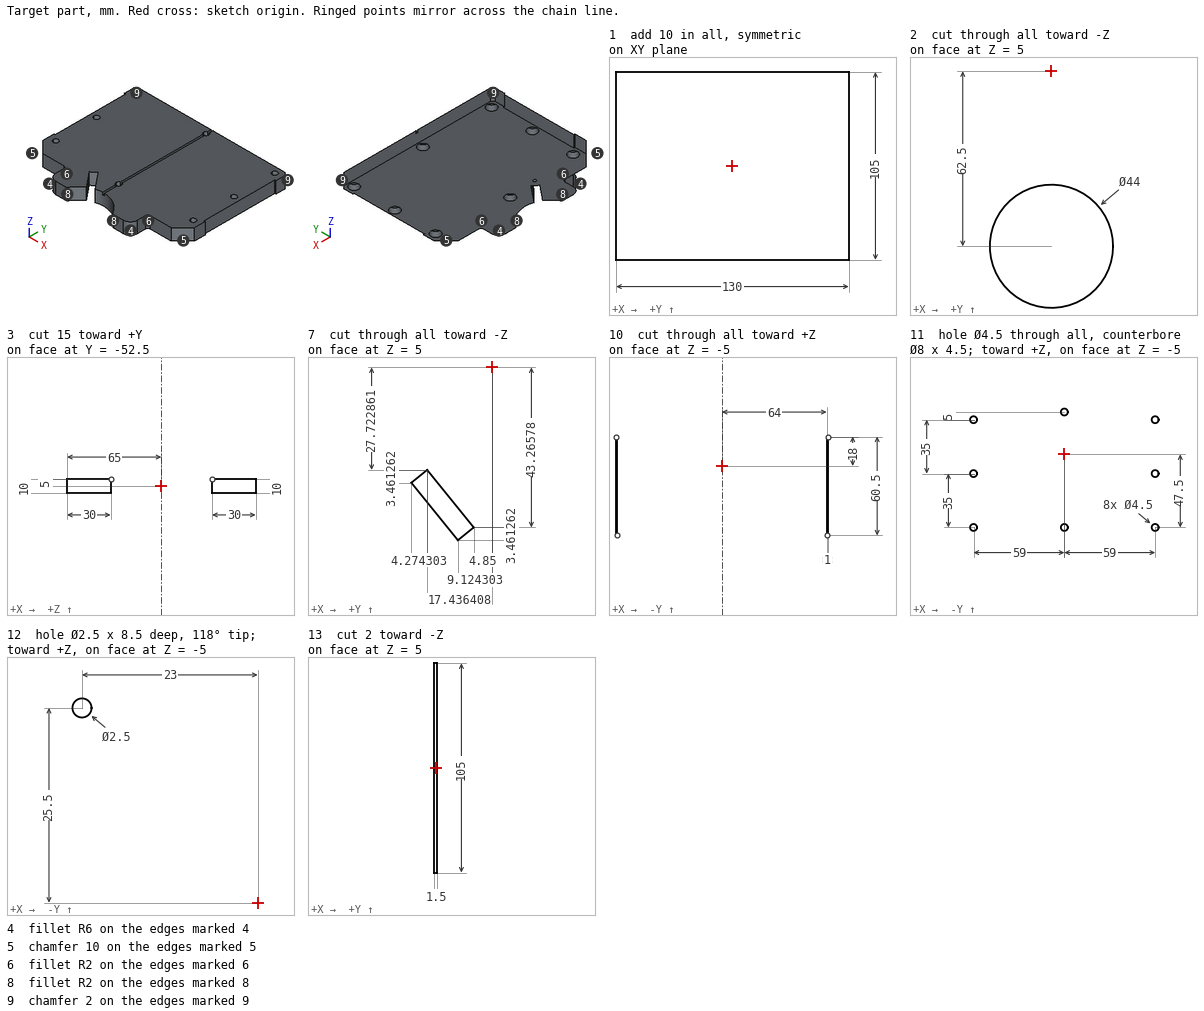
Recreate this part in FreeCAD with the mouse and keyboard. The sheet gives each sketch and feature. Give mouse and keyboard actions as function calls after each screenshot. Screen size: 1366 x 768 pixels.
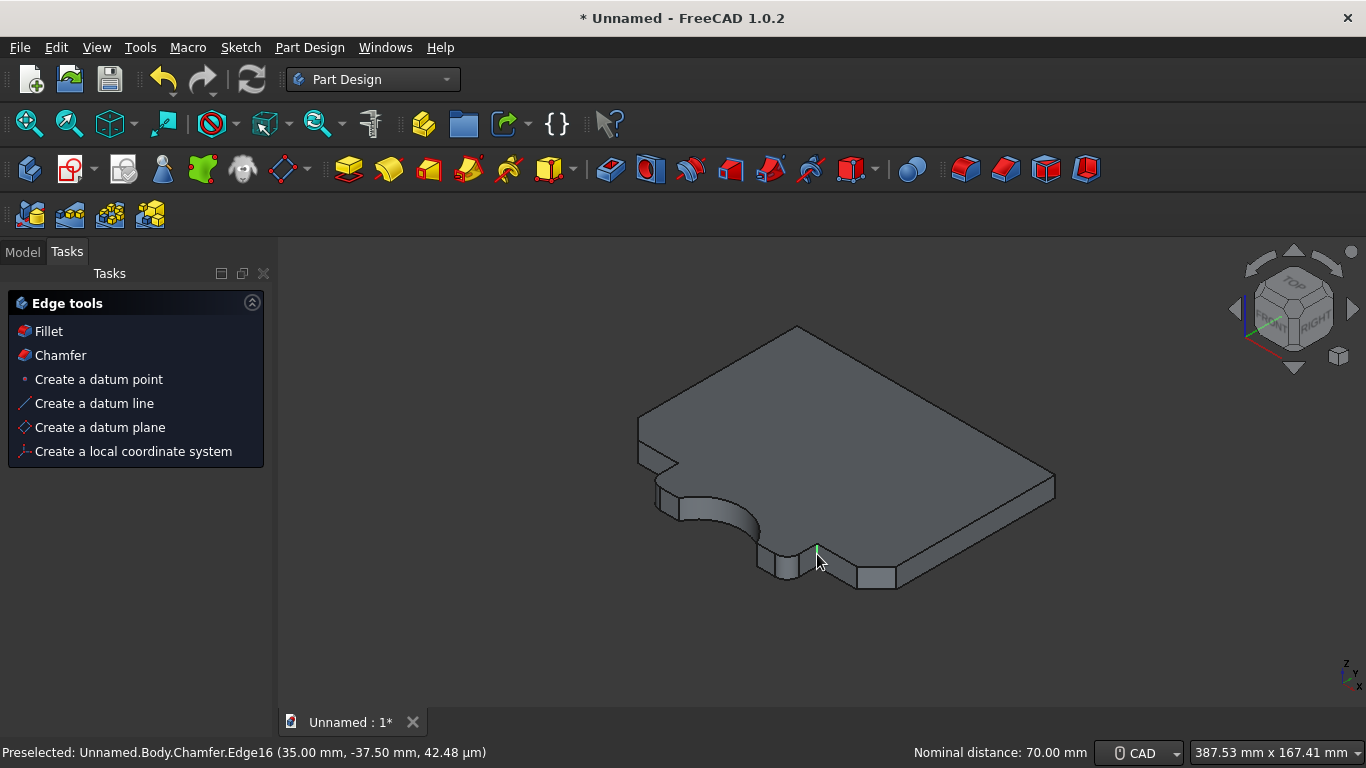
click(966, 170)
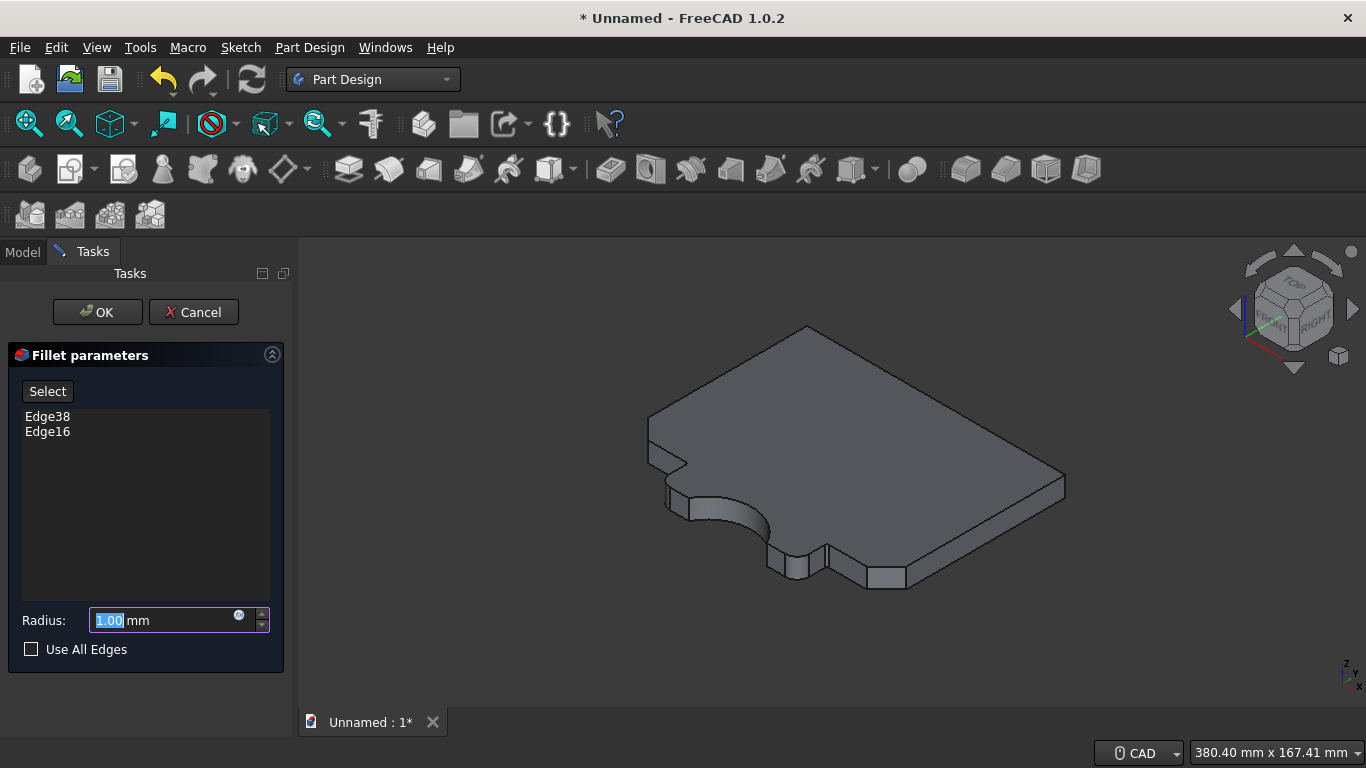
text(2)
key(Tab)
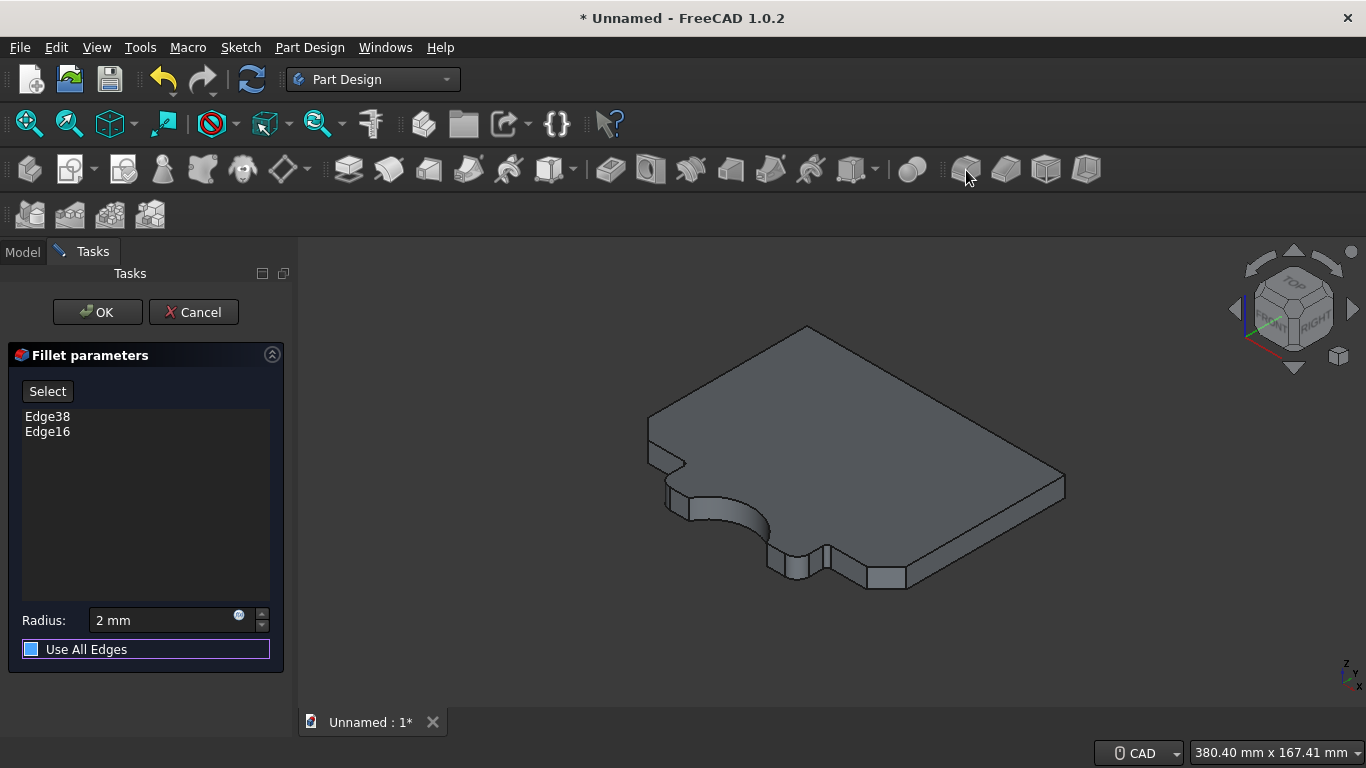
click(98, 312)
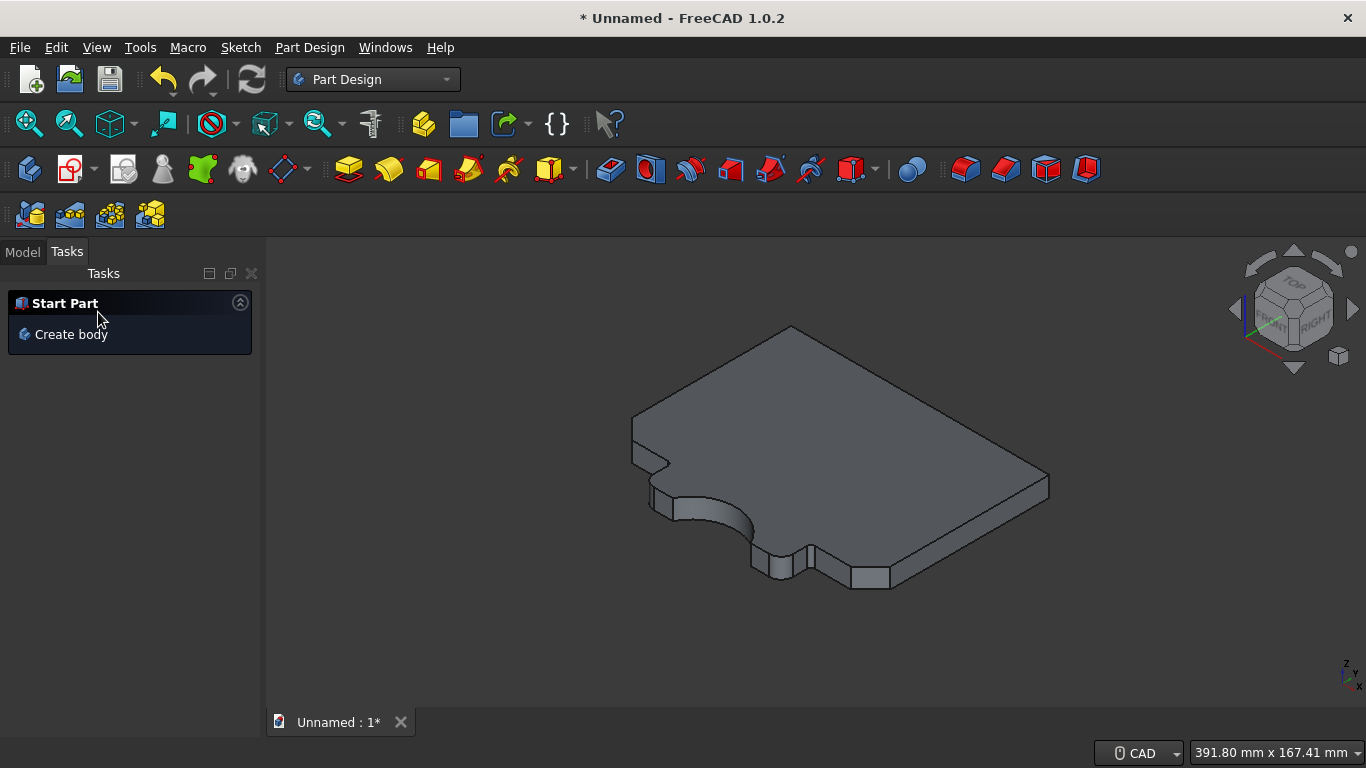
click(779, 438)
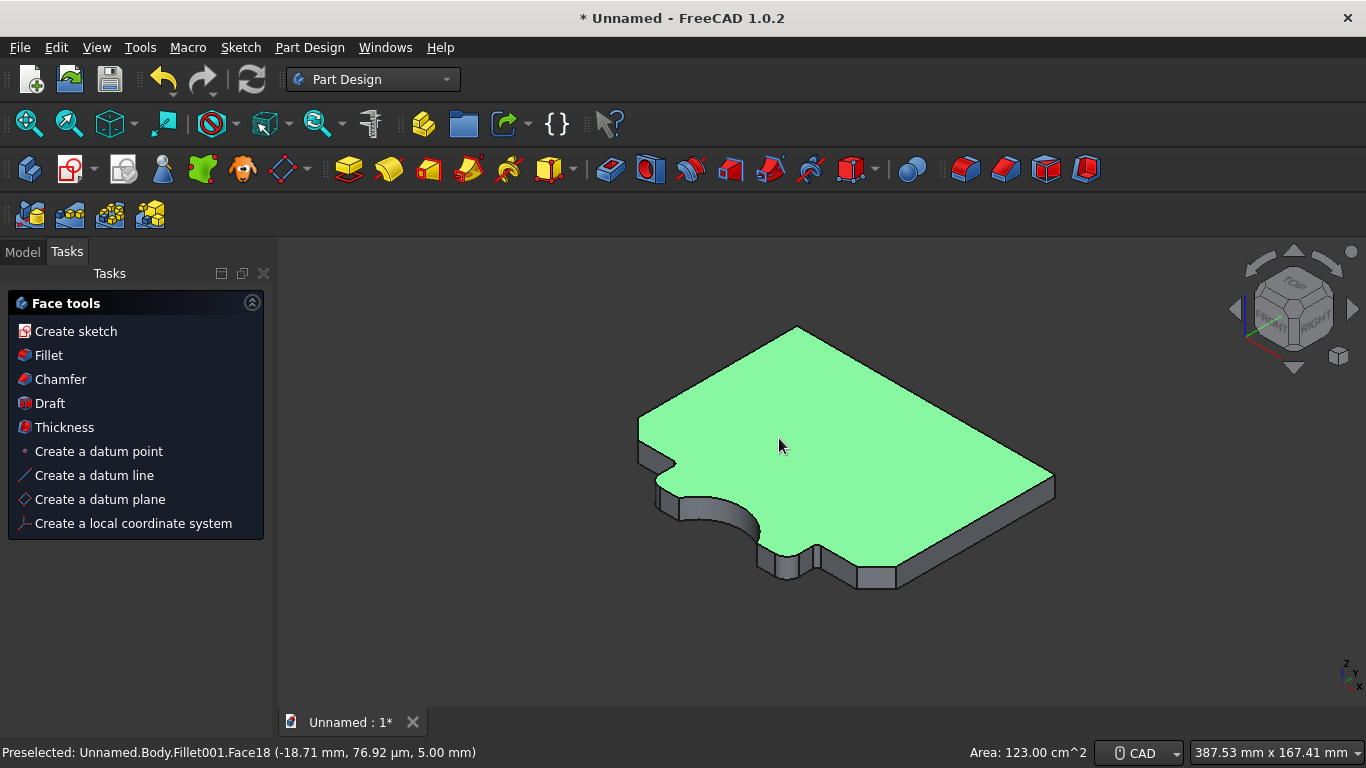
click(70, 170)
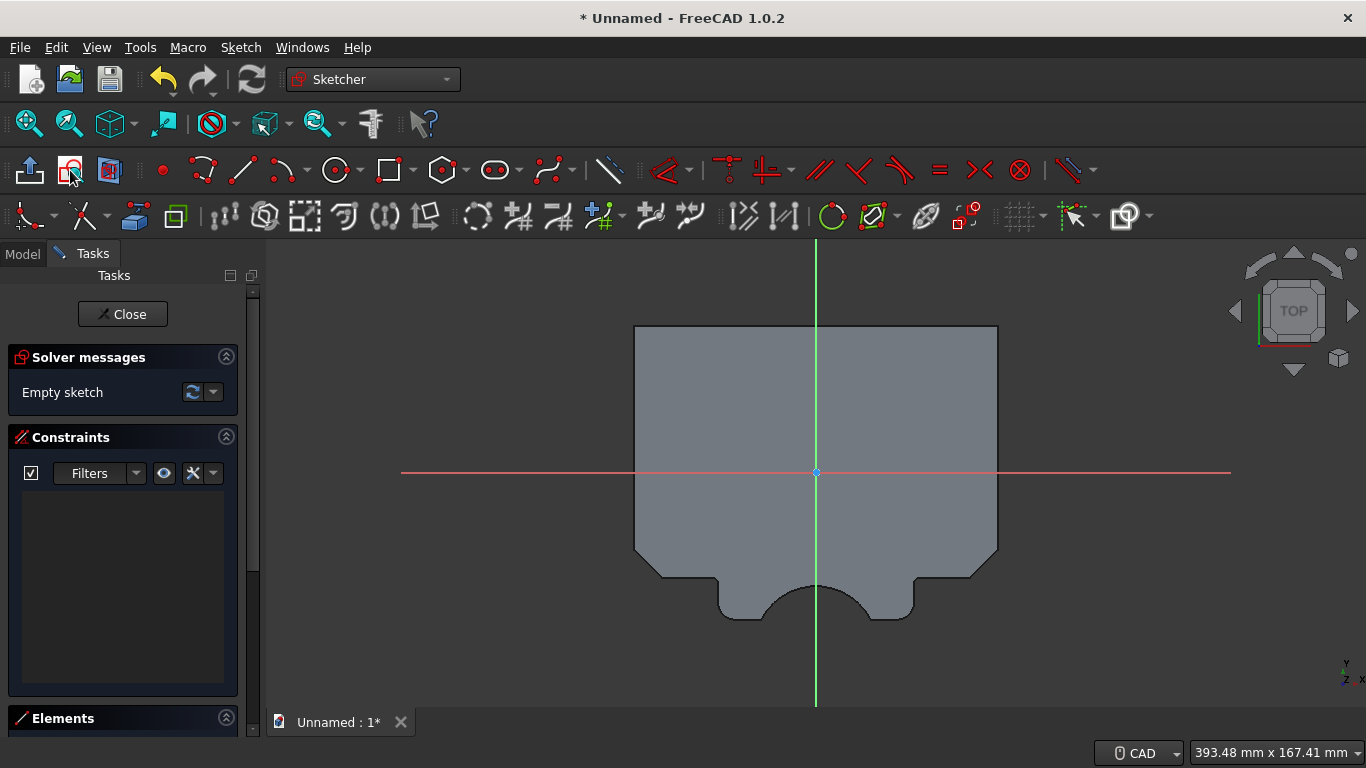
scroll(817, 592, up, 4)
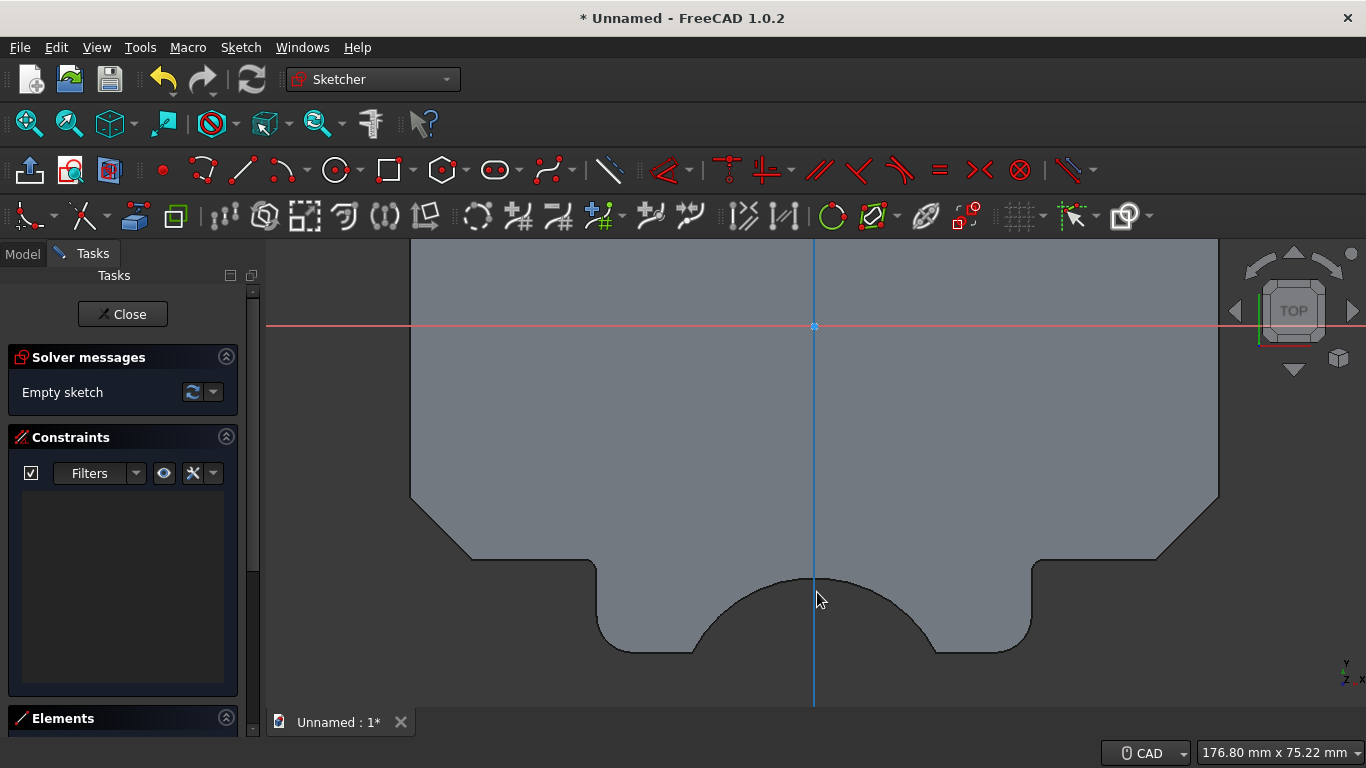
click(204, 170)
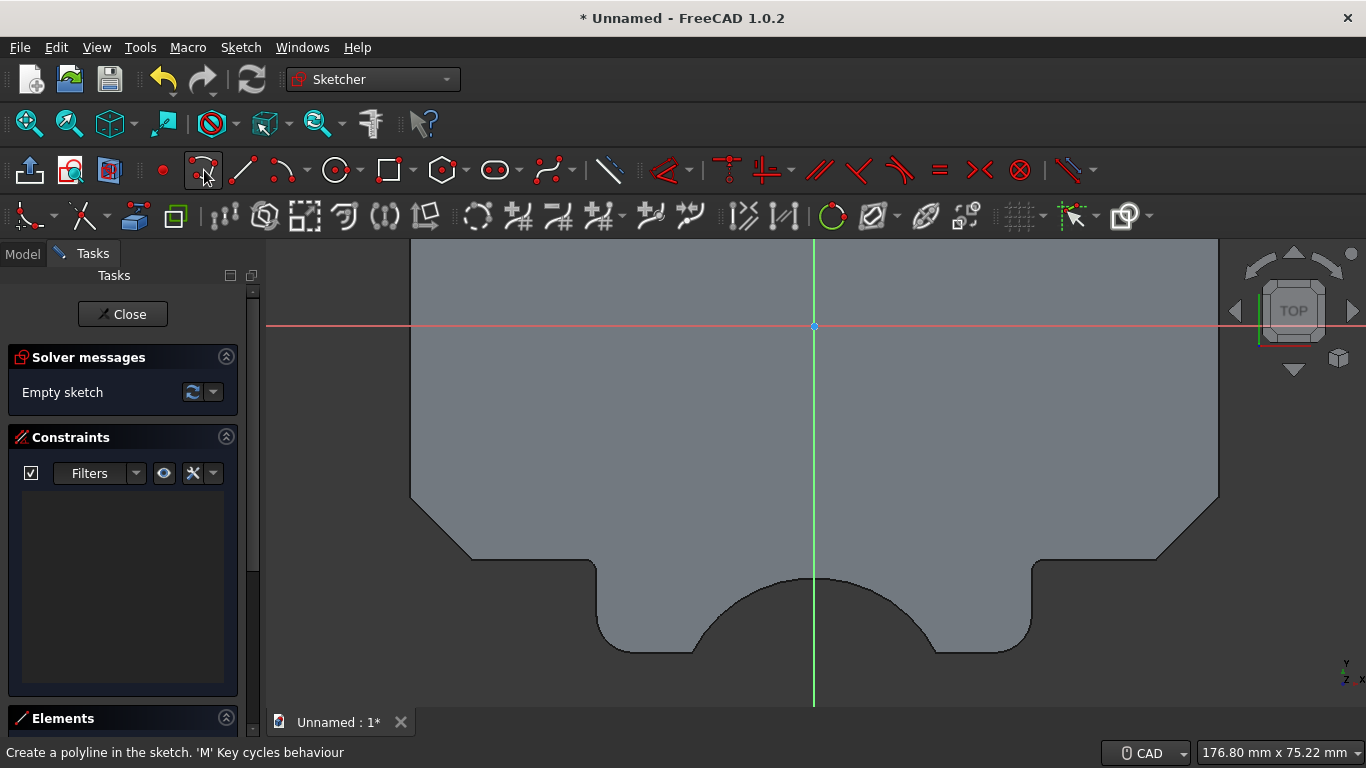
click(706, 499)
click(679, 520)
click(757, 617)
click(784, 595)
click(706, 500)
key(Escape)
key(Escape)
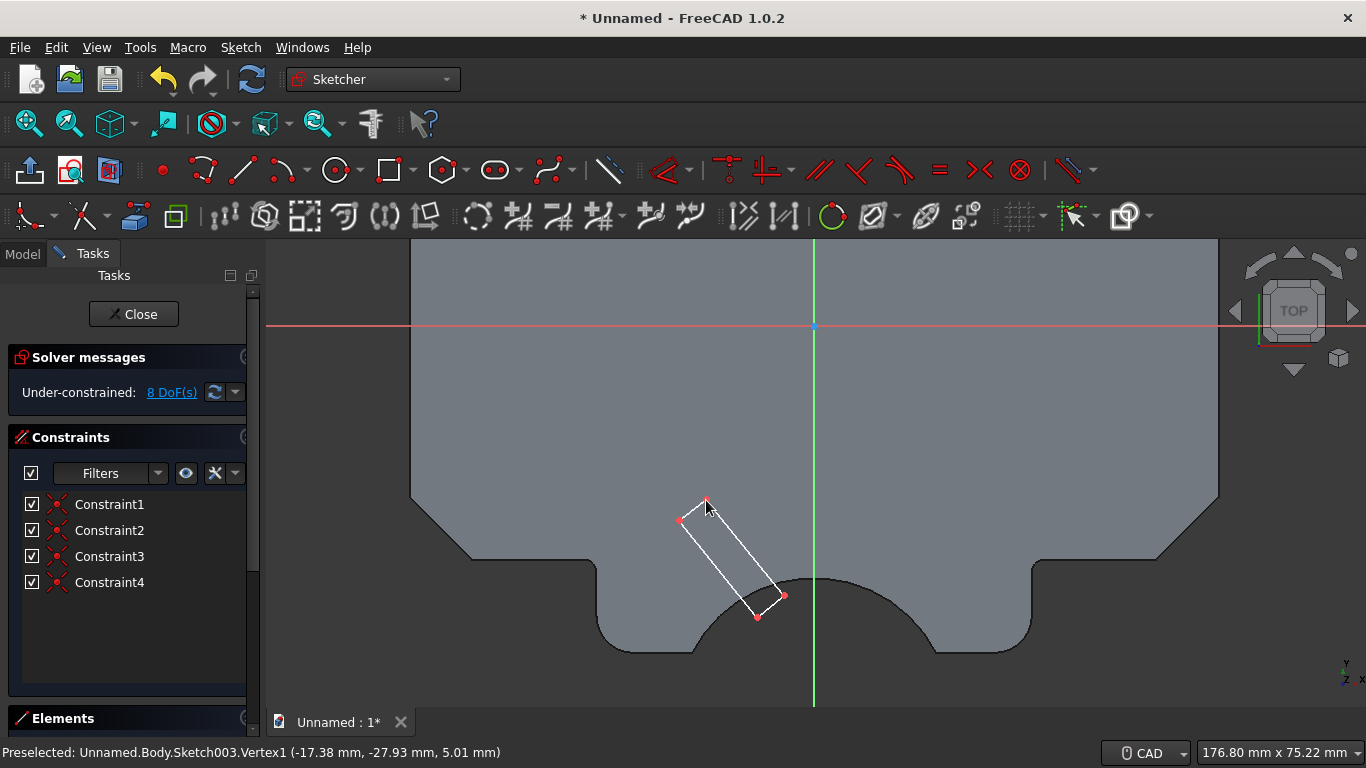
click(664, 170)